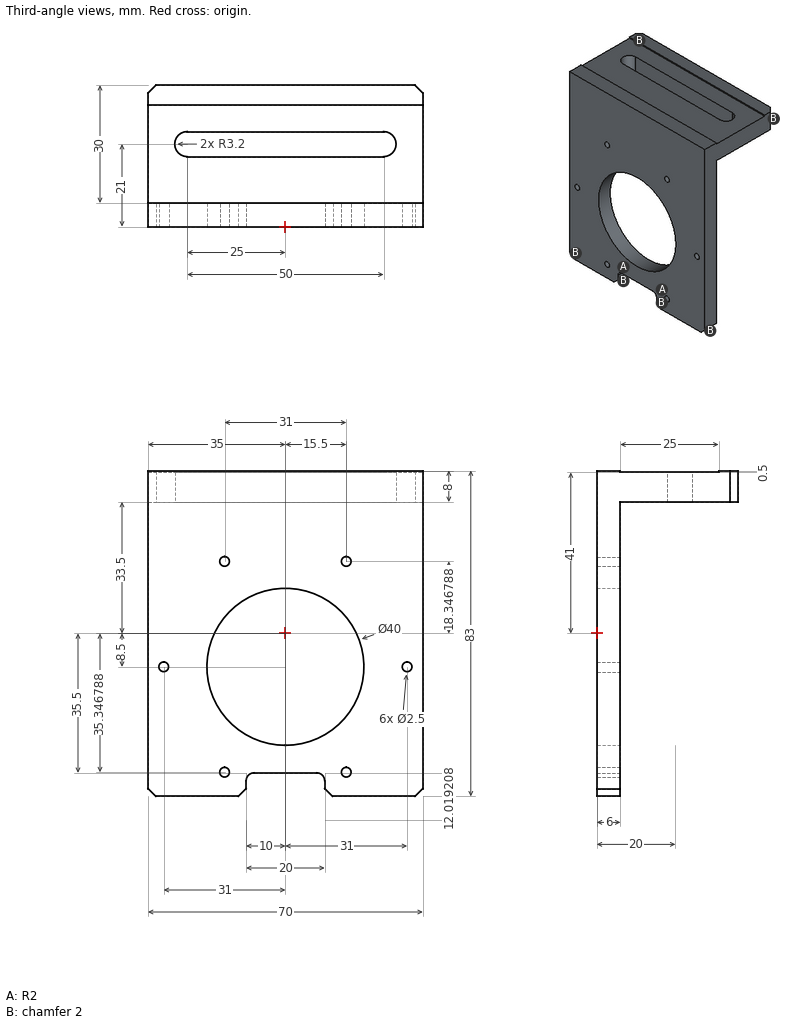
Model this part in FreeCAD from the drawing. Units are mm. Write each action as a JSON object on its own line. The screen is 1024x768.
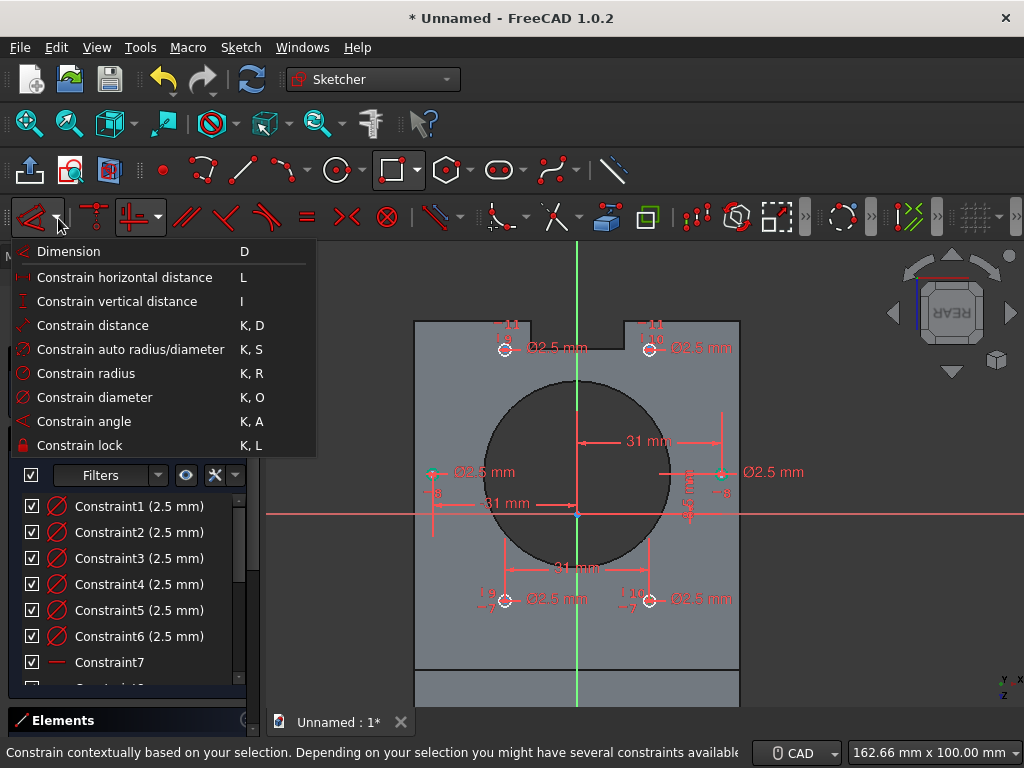
{"action": "left_click", "coordinate": [164, 277]}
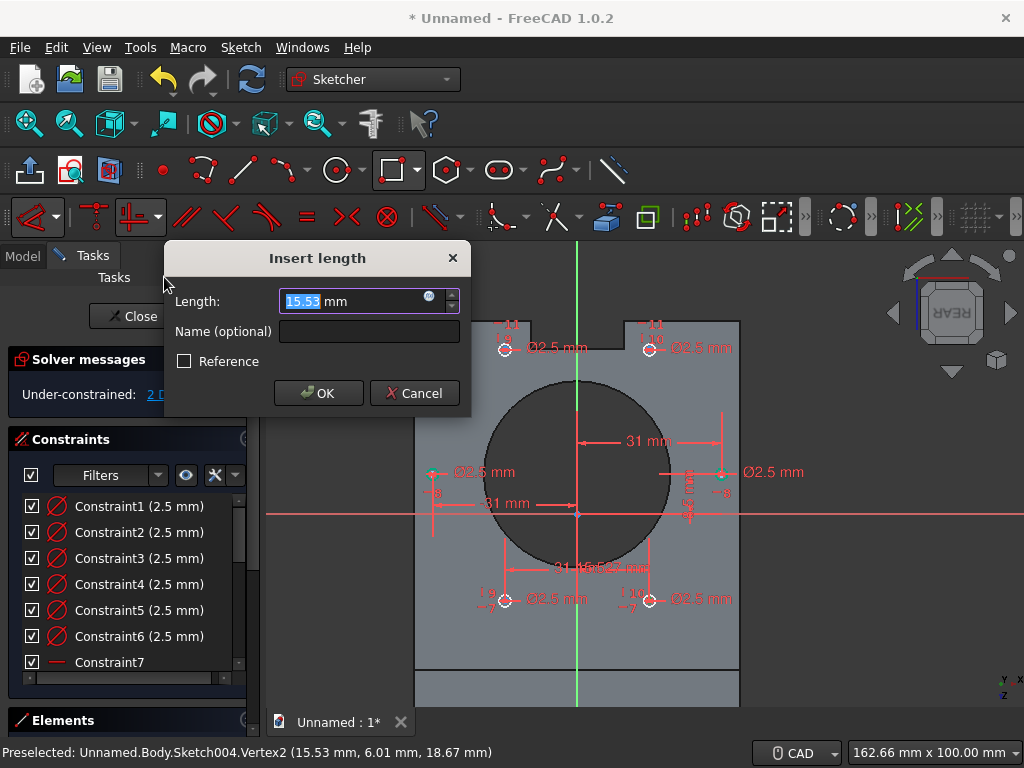
{"action": "type", "text": "15.5"}
{"action": "key", "text": "Return"}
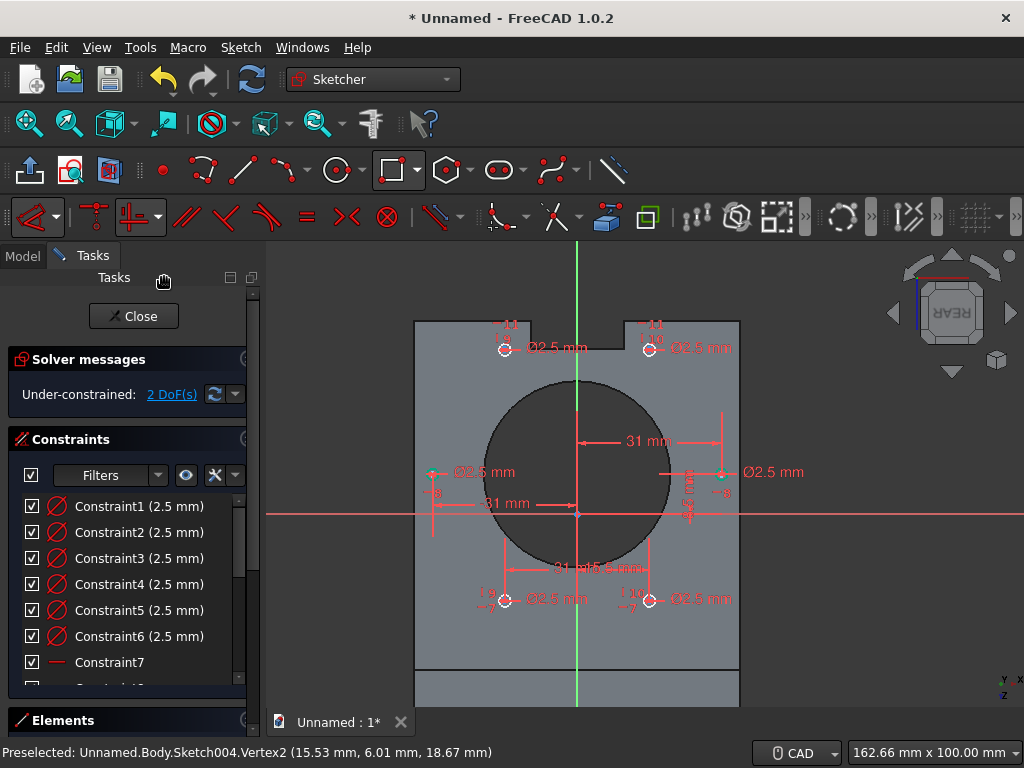
{"action": "left_click", "coordinate": [649, 601]}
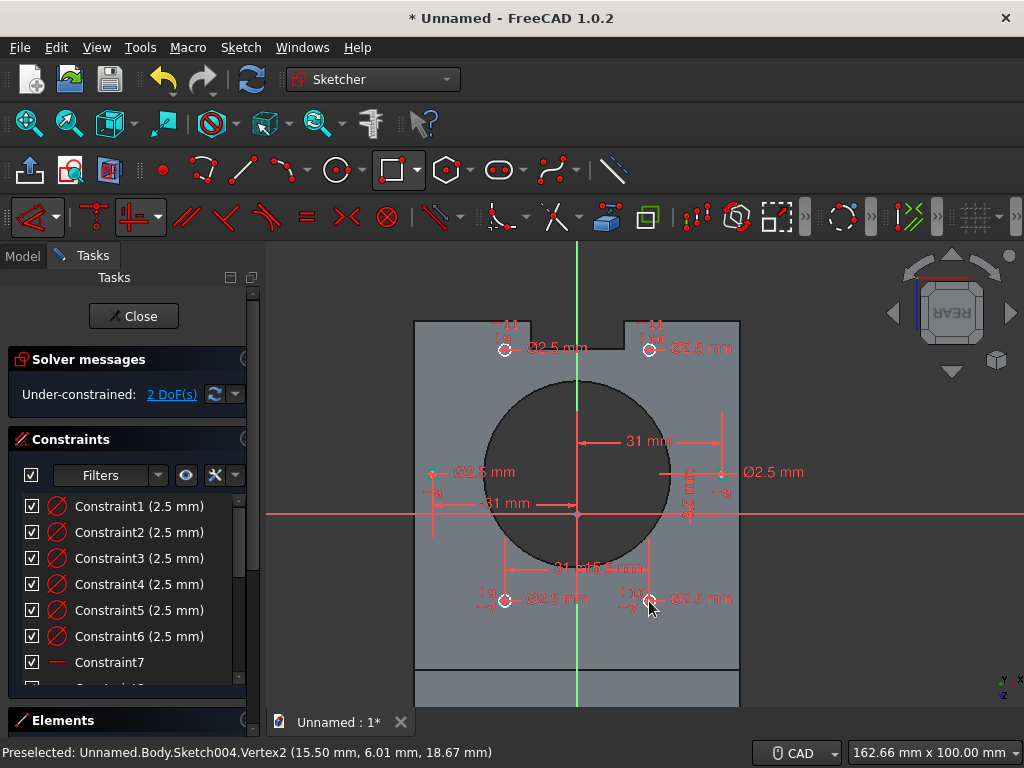
{"action": "left_click", "coordinate": [58, 218]}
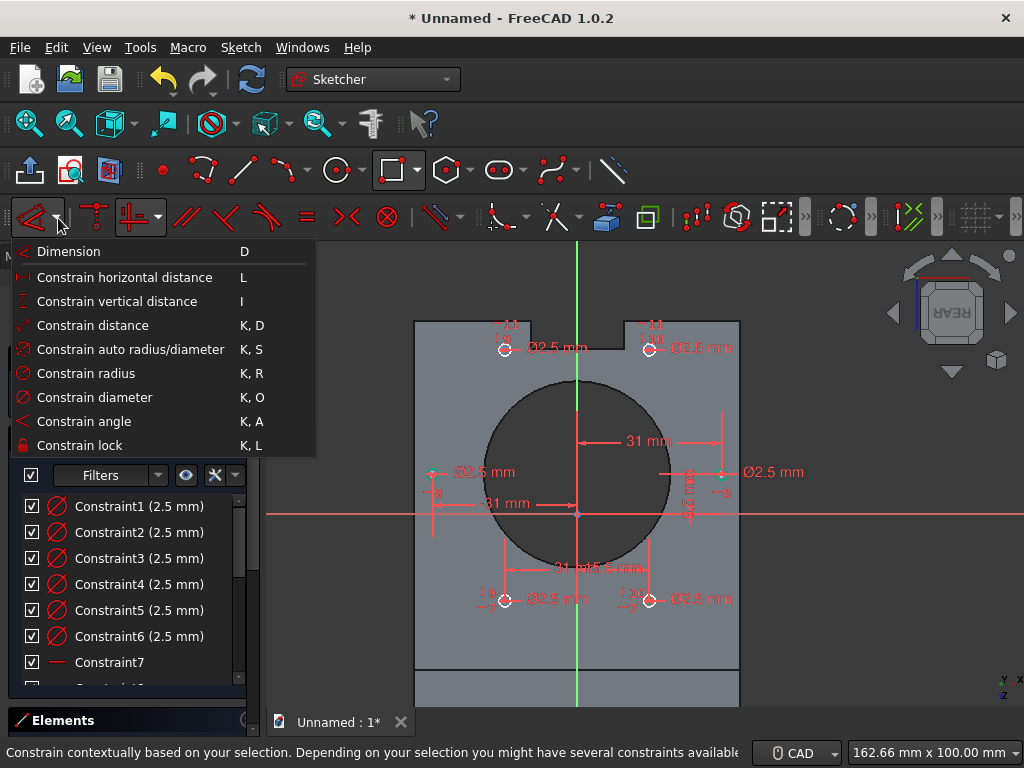
{"action": "left_click", "coordinate": [164, 301]}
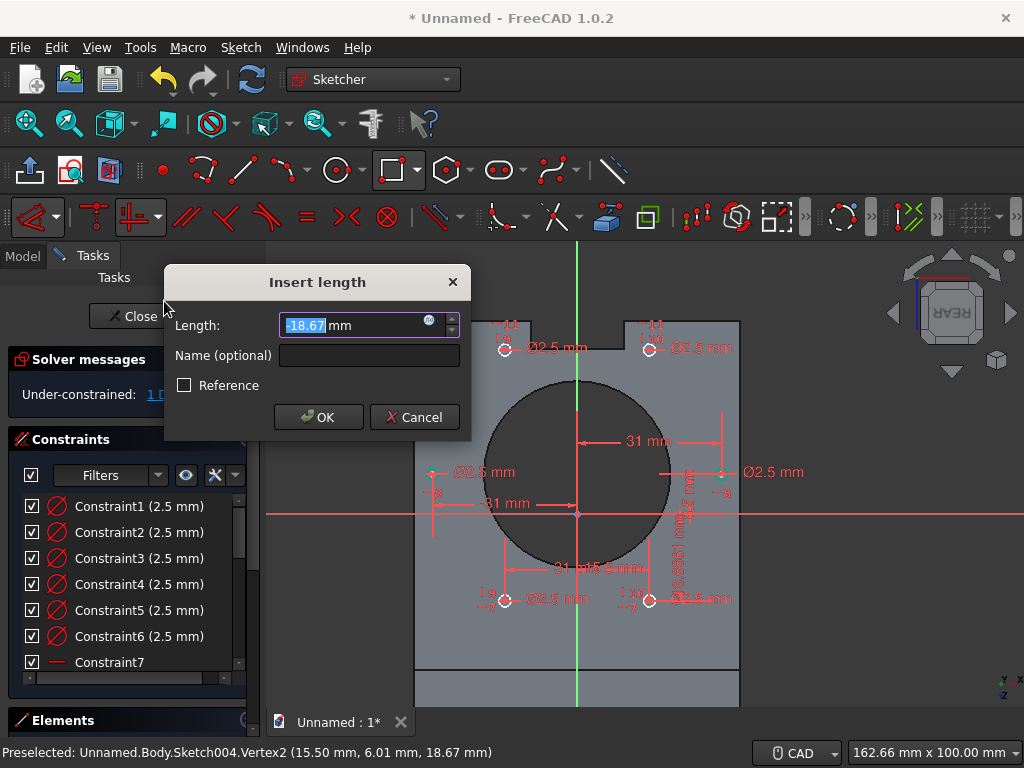
{"action": "type", "text": "-18.346788"}
{"action": "key", "text": "Return"}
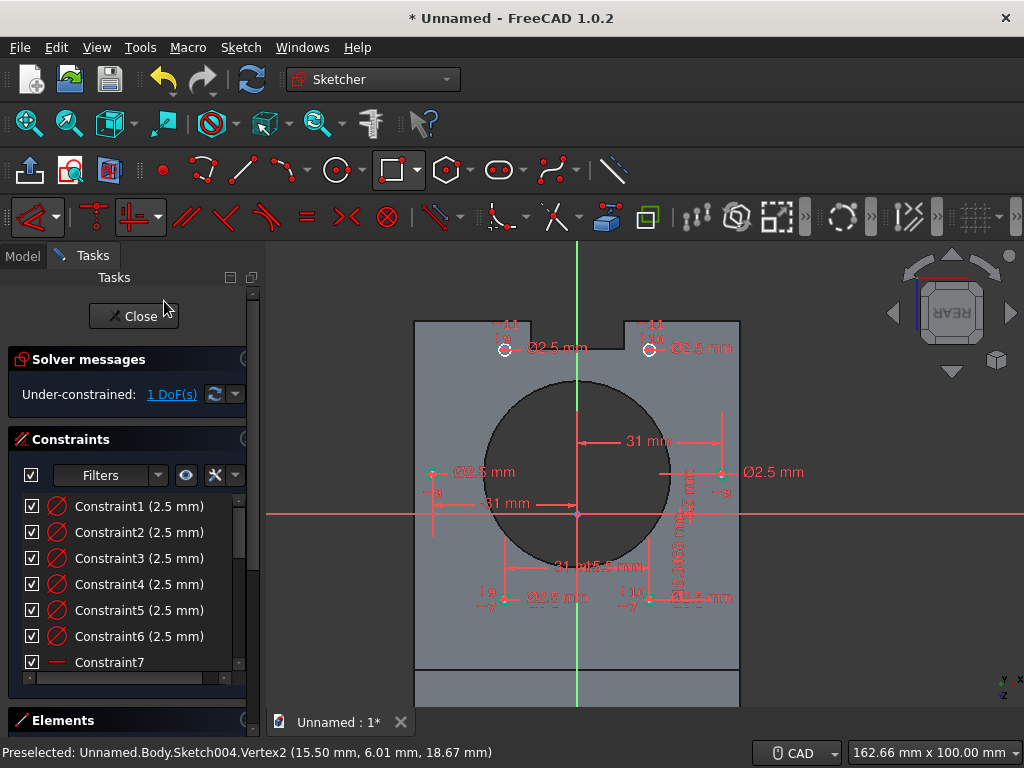
{"action": "left_click", "coordinate": [505, 350]}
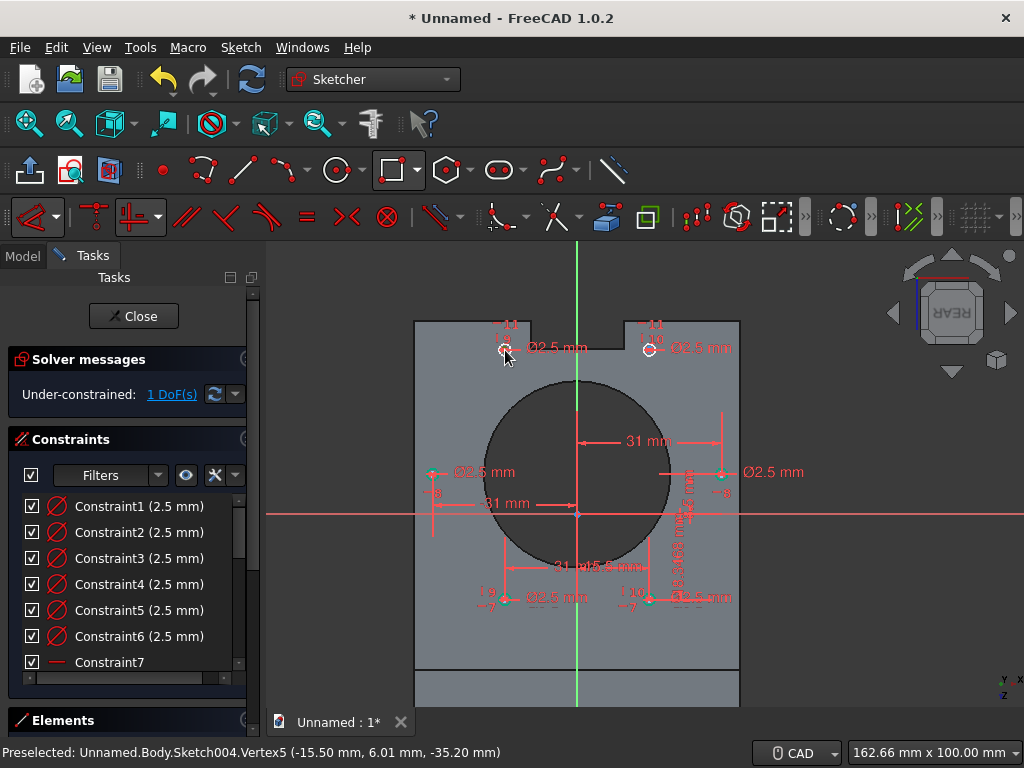
{"action": "left_click", "coordinate": [58, 218]}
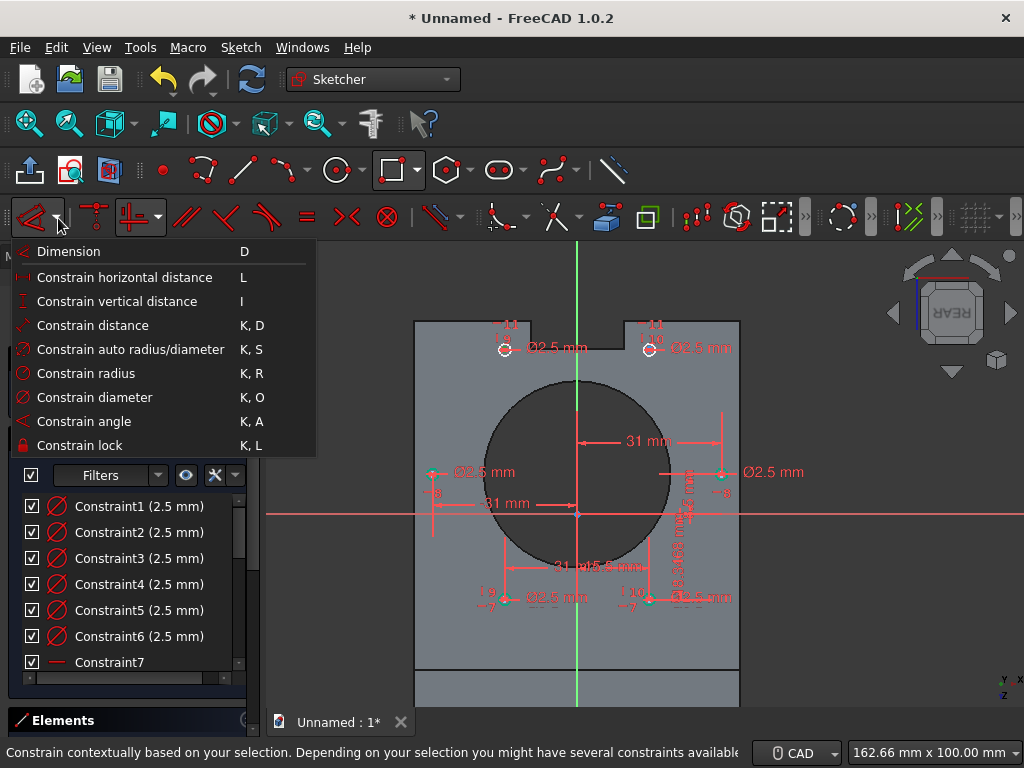
{"action": "left_click", "coordinate": [164, 301]}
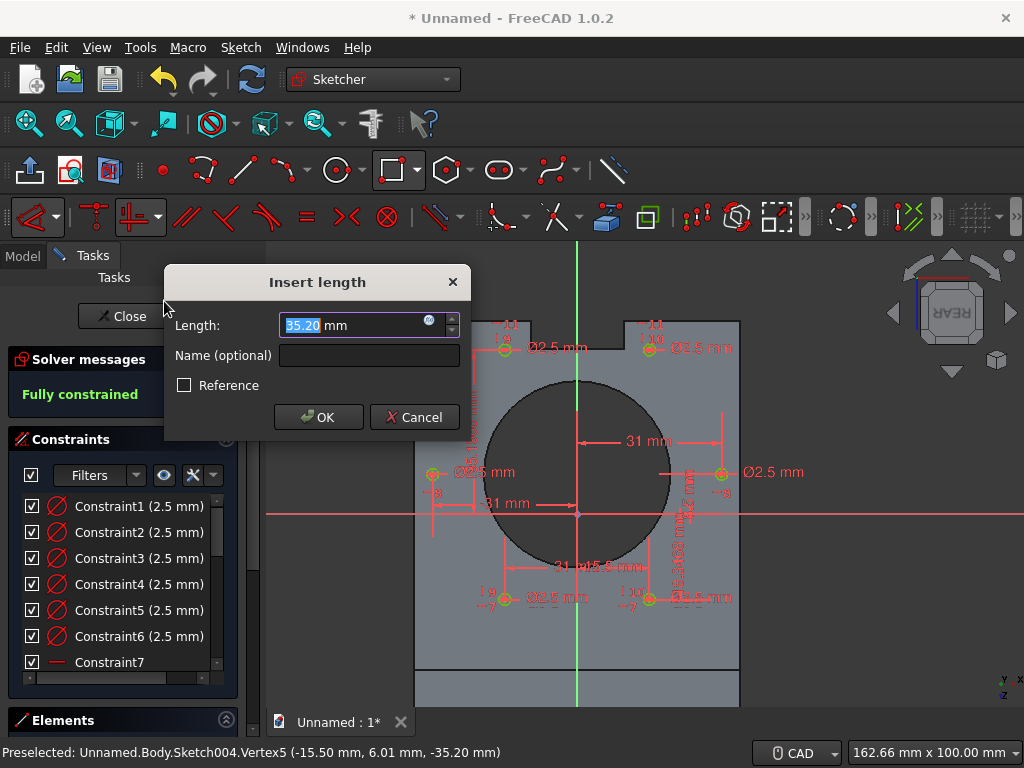
{"action": "type", "text": "35.346788"}
{"action": "key", "text": "Return"}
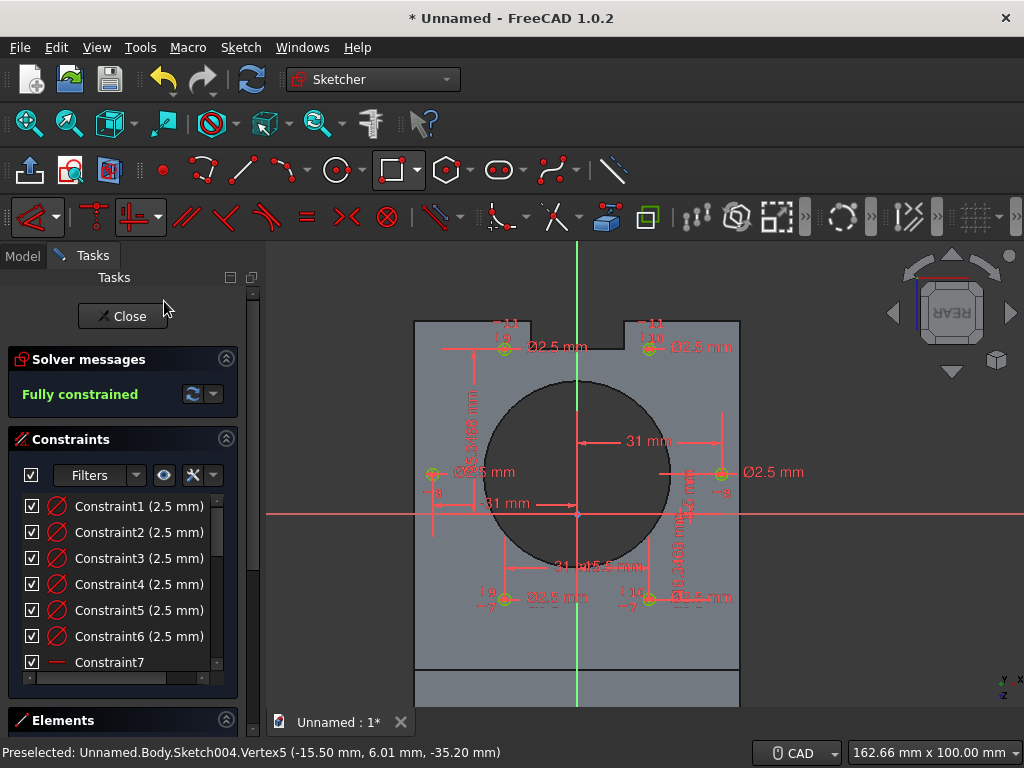
{"action": "left_click", "coordinate": [123, 316]}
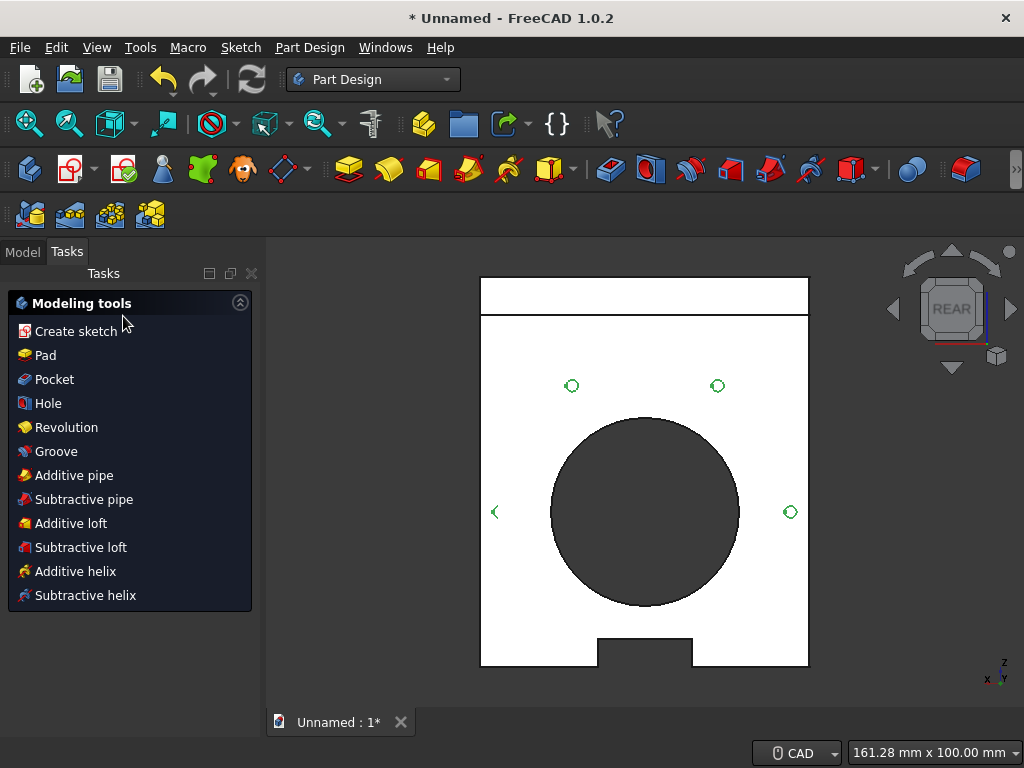
{"action": "left_click", "coordinate": [612, 170]}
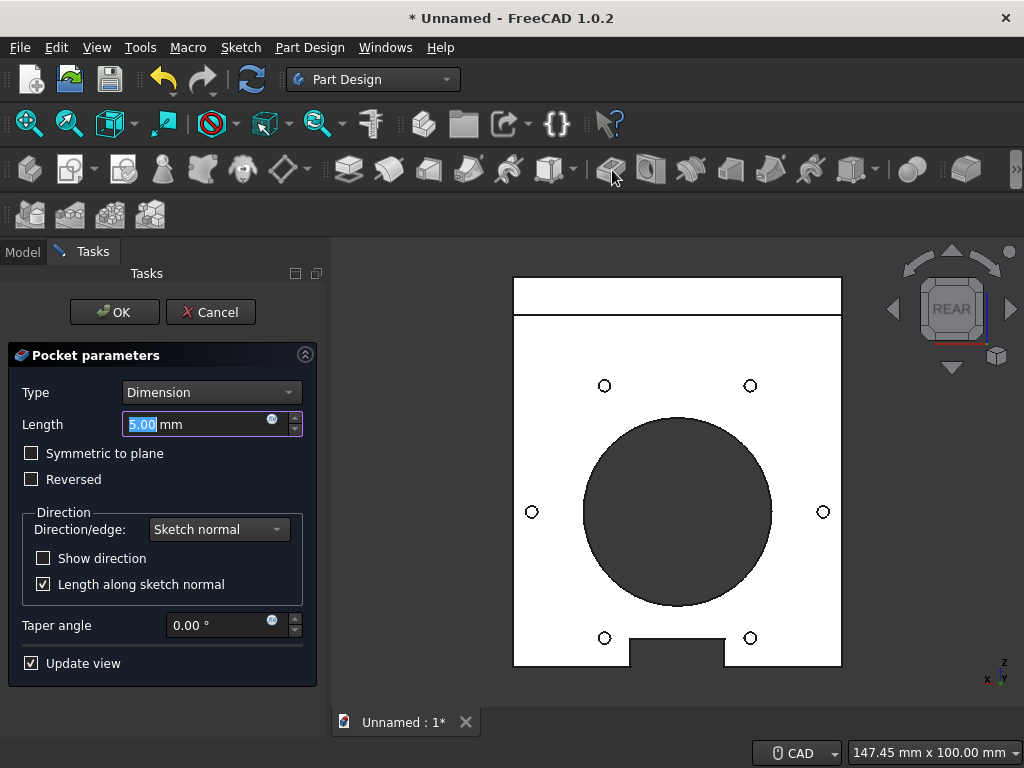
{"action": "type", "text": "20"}
{"action": "key", "text": "Tab"}